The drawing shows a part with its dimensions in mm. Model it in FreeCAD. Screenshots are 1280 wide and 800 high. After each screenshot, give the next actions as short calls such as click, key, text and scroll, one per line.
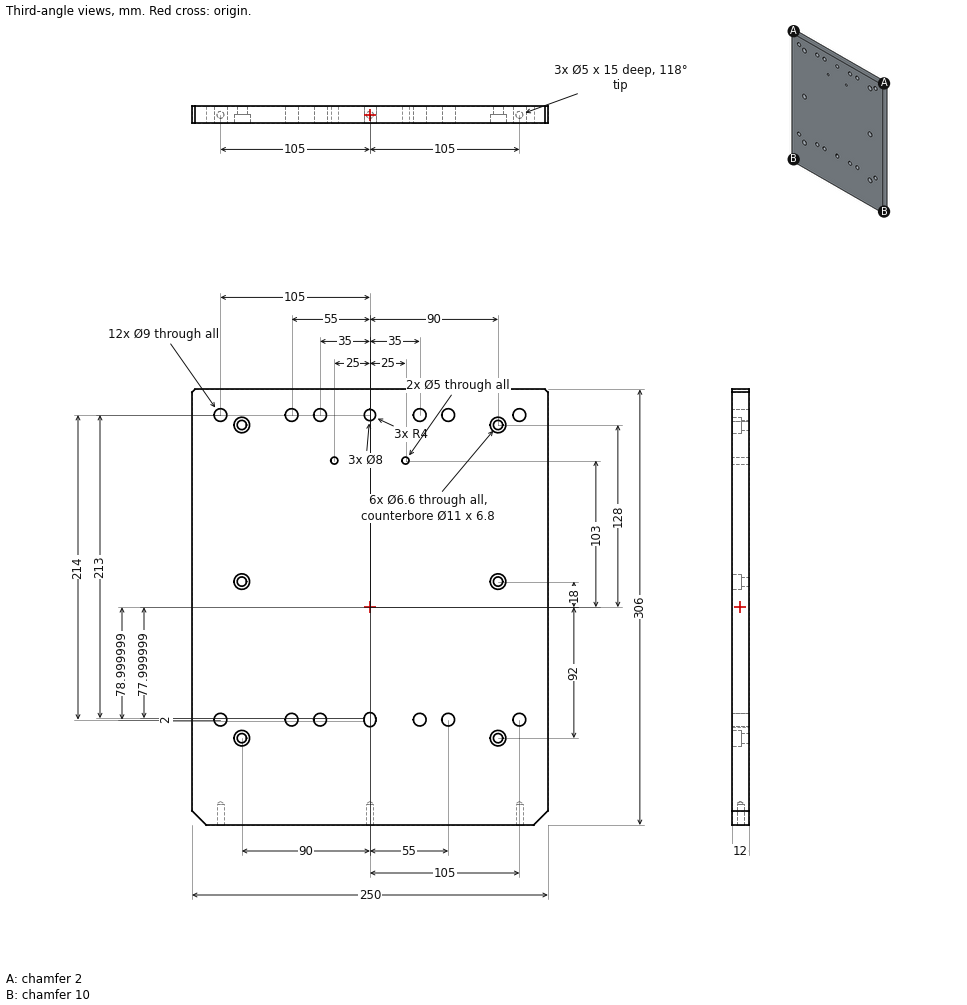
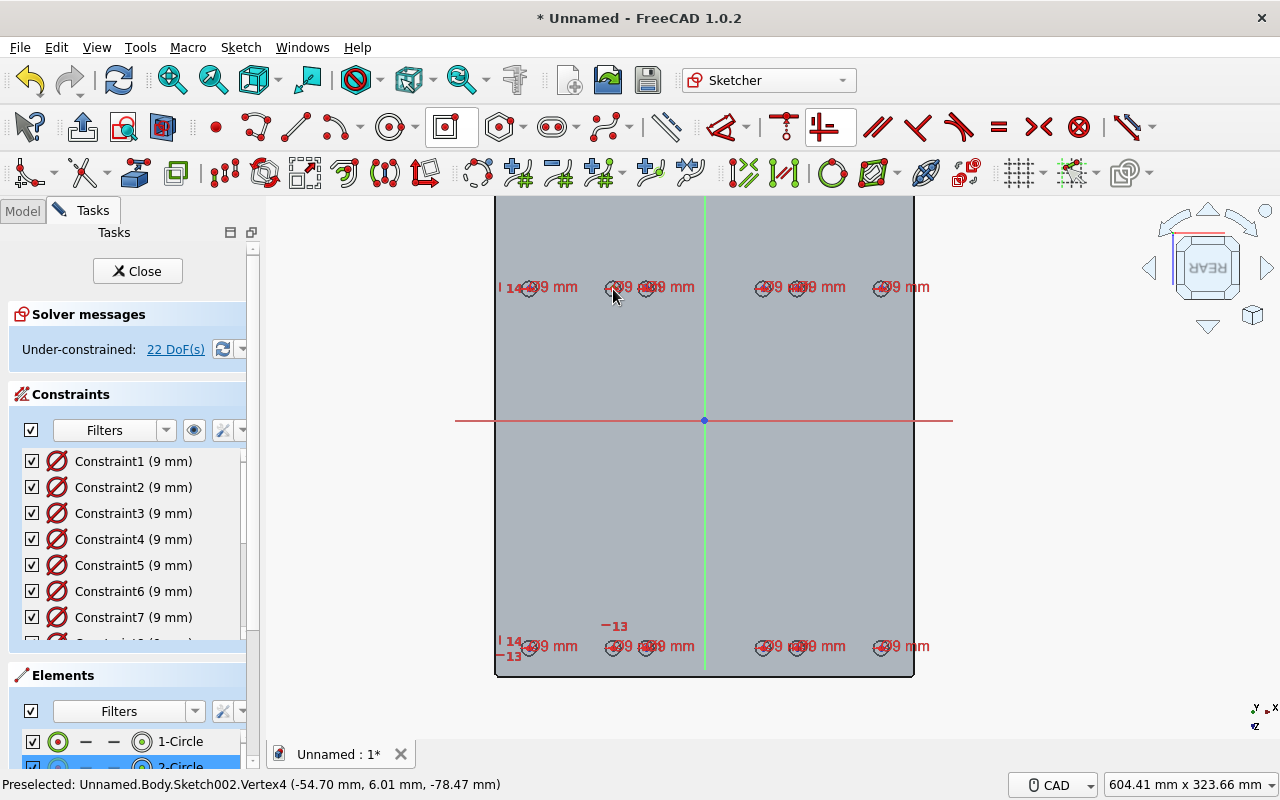
click(850, 128)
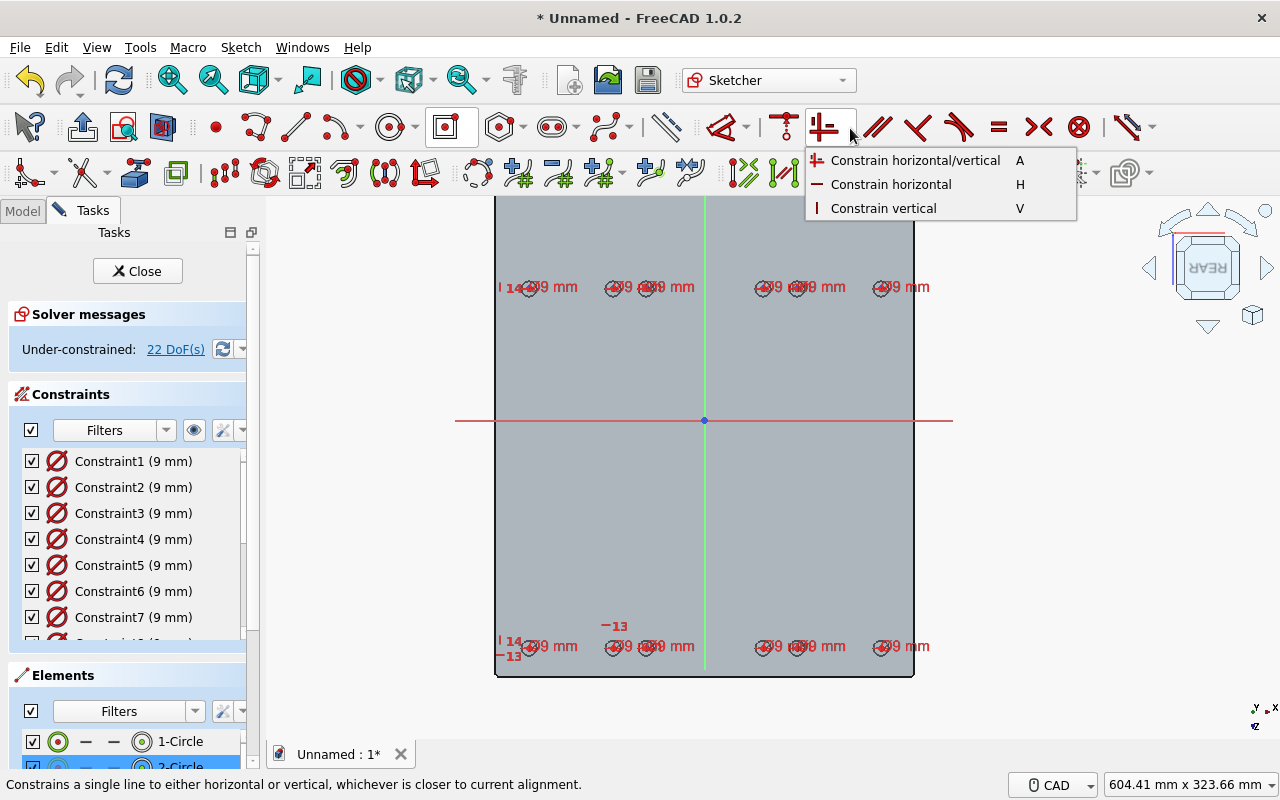
click(941, 208)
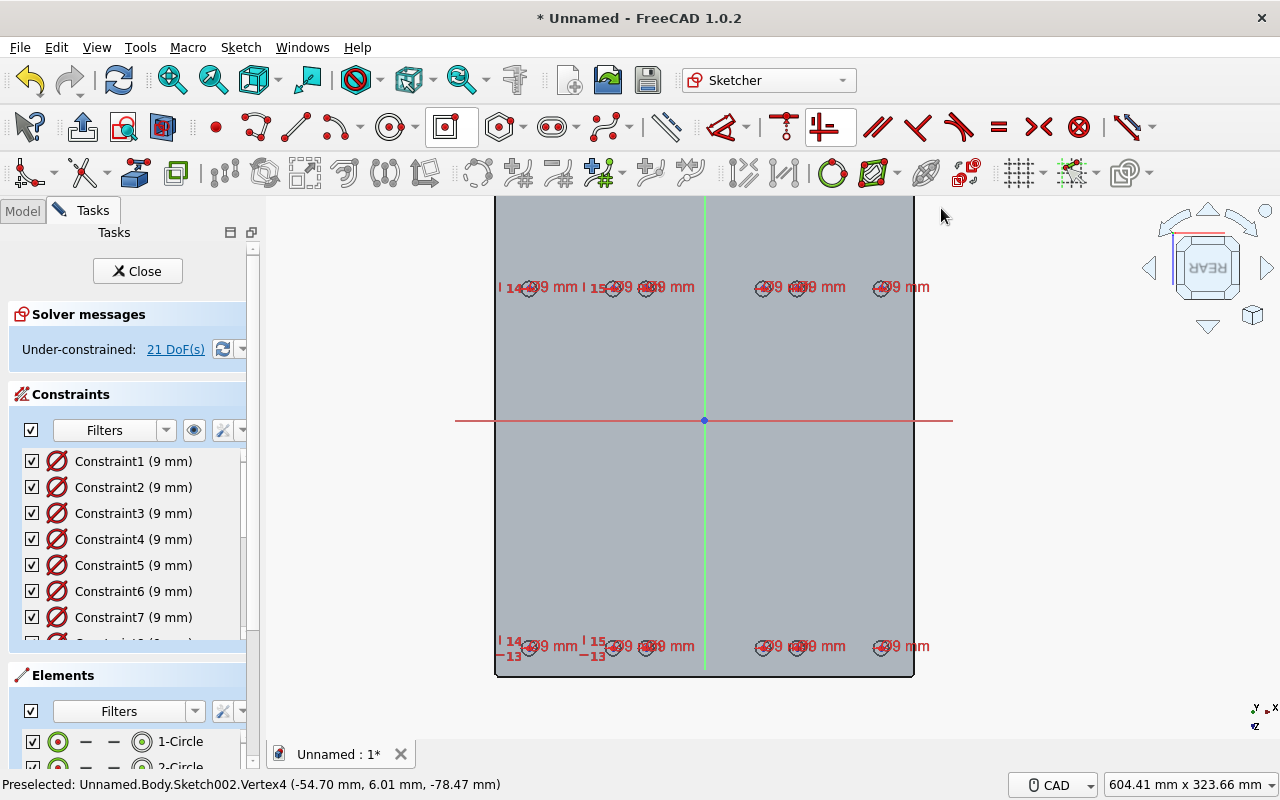
click(529, 289)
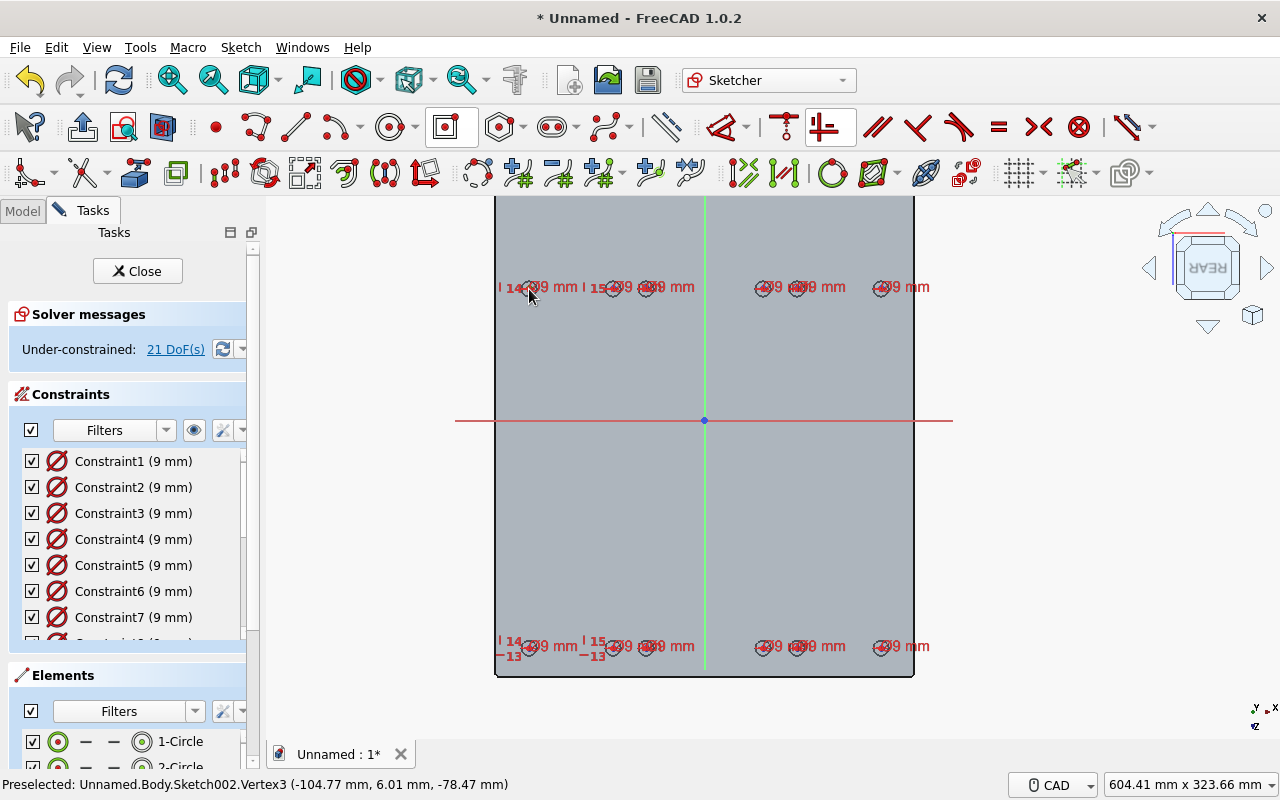
click(613, 289)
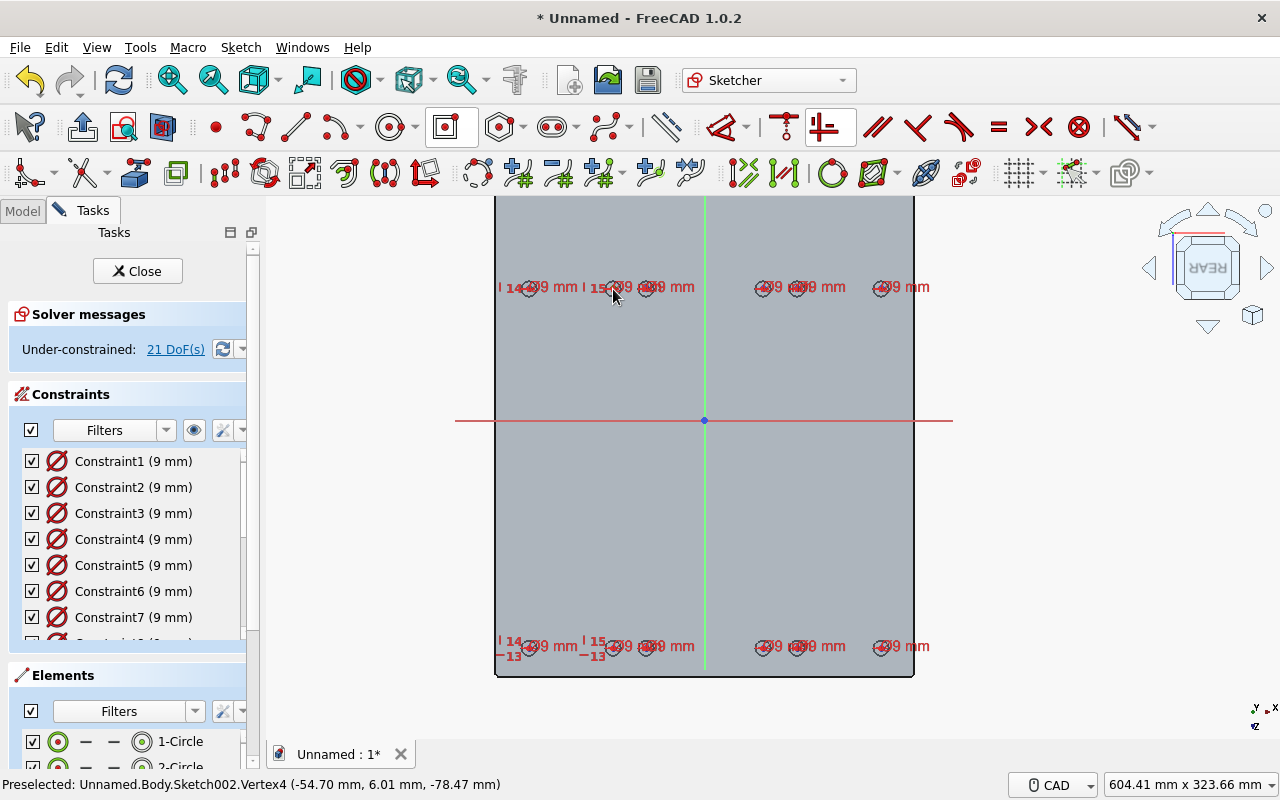
key(h)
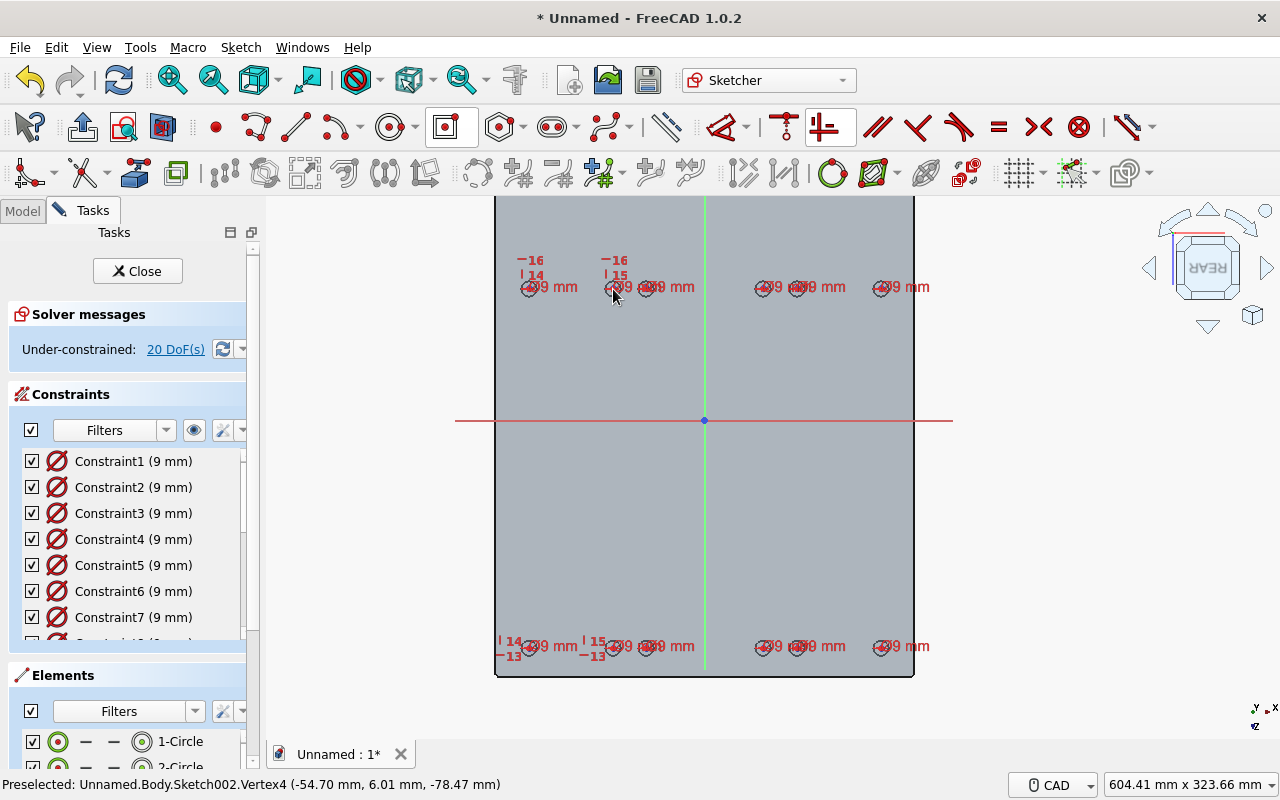
click(613, 289)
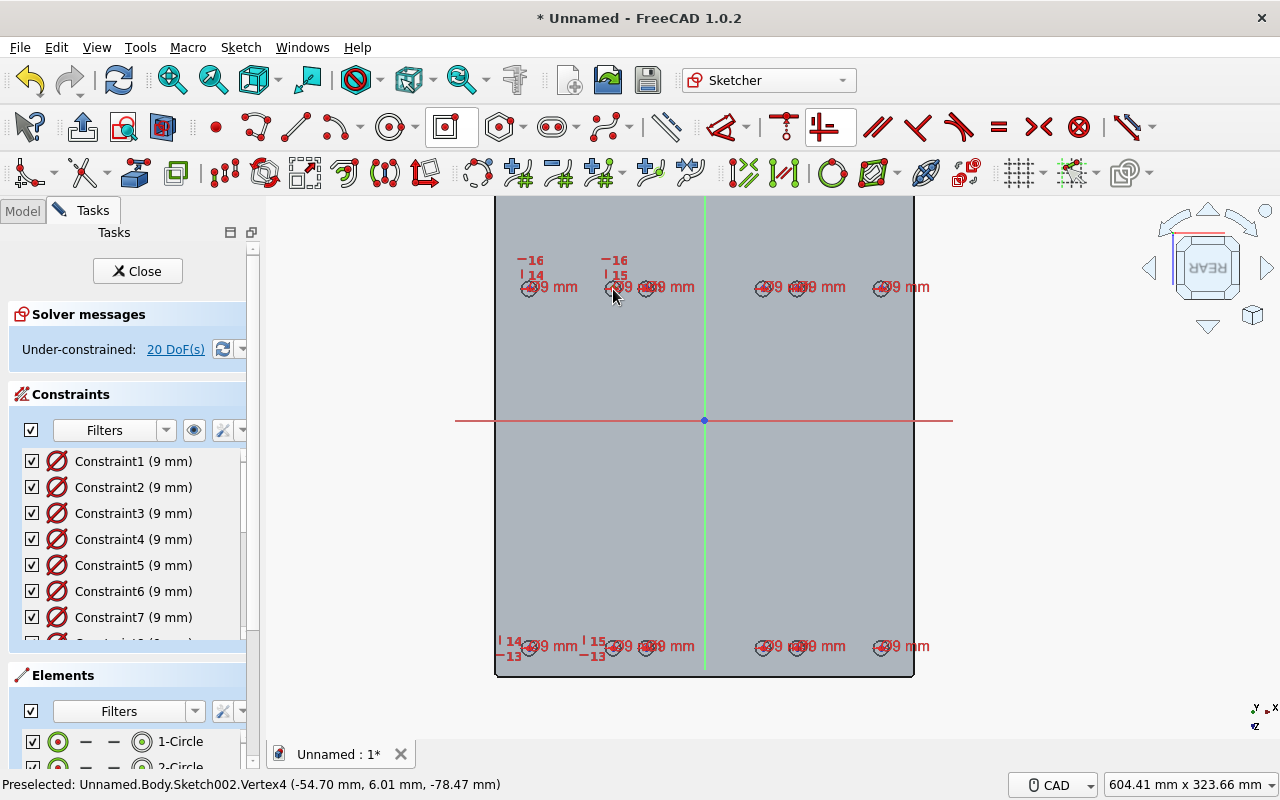
click(797, 289)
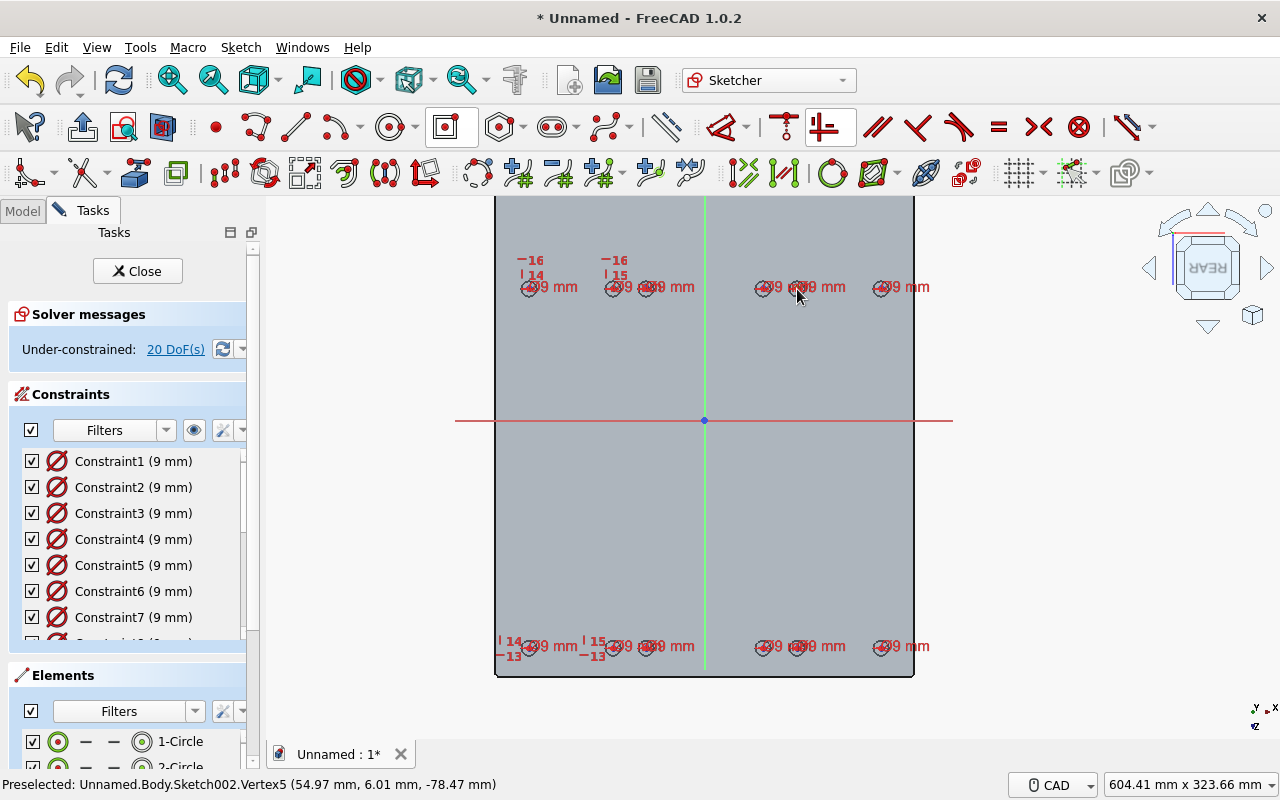
click(850, 128)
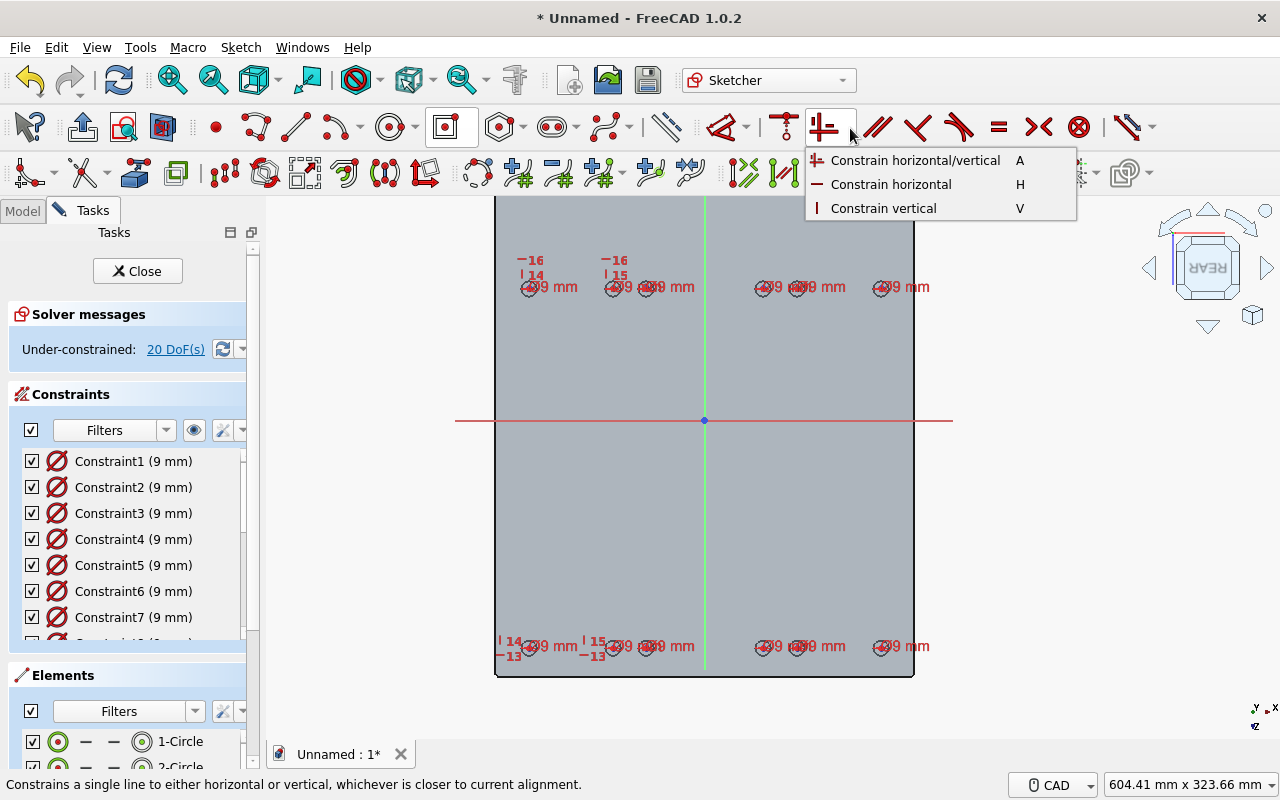
click(941, 184)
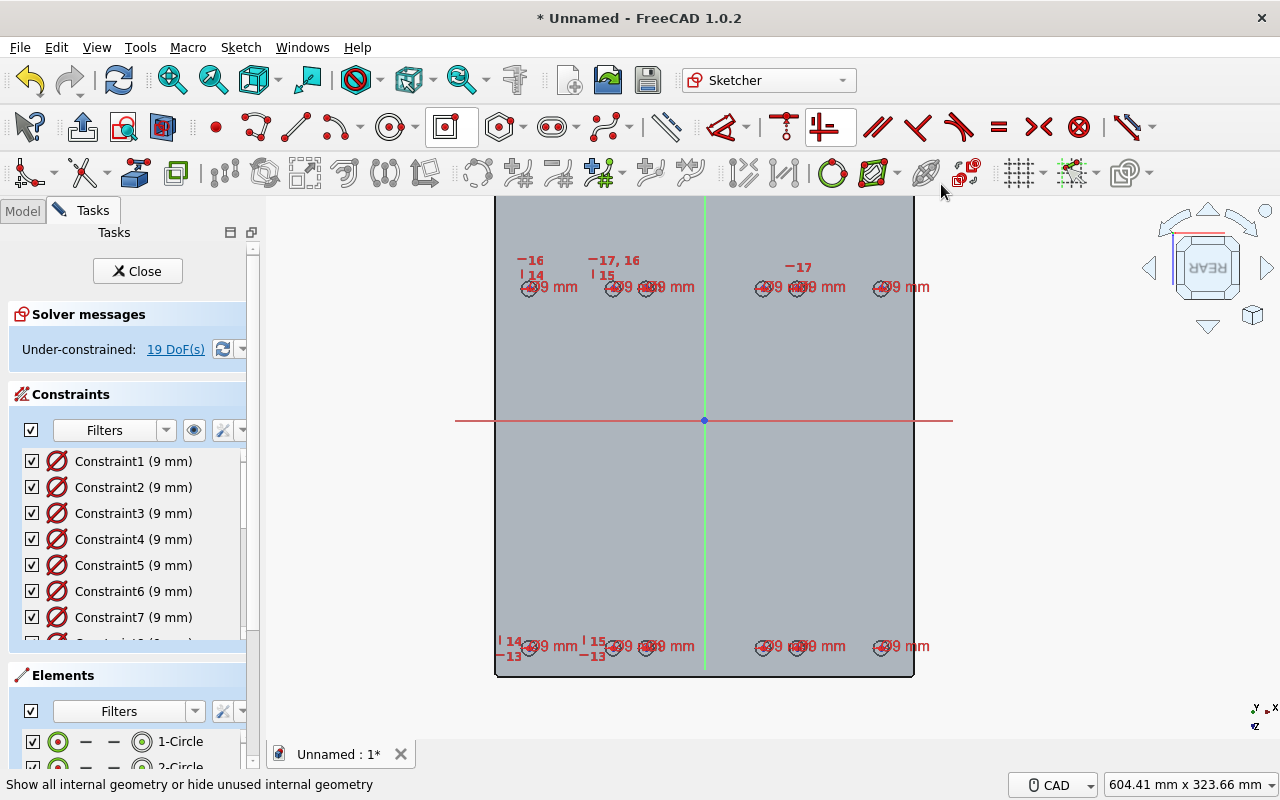
click(797, 289)